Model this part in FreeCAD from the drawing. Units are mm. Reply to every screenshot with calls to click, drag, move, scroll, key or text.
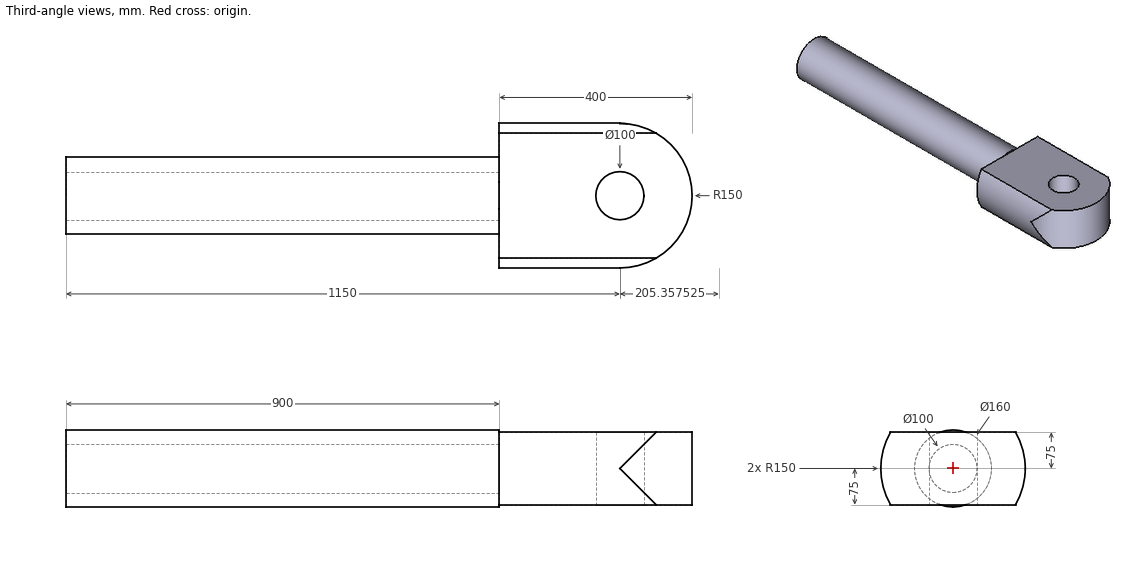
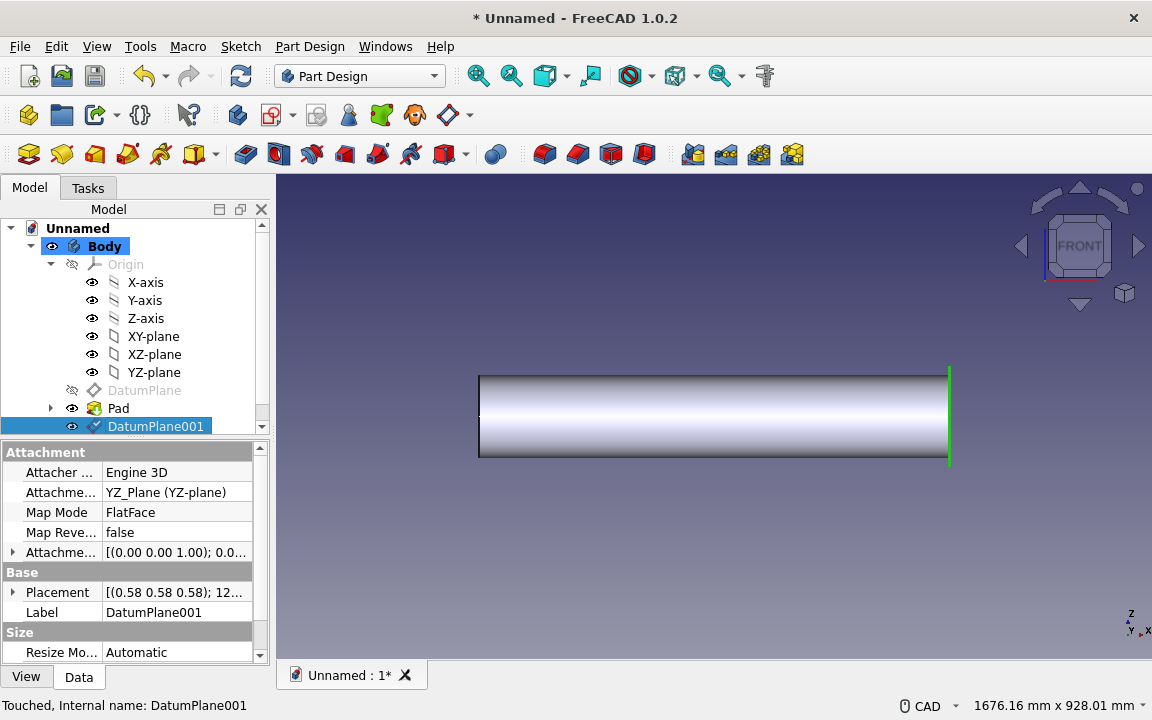
click(270, 116)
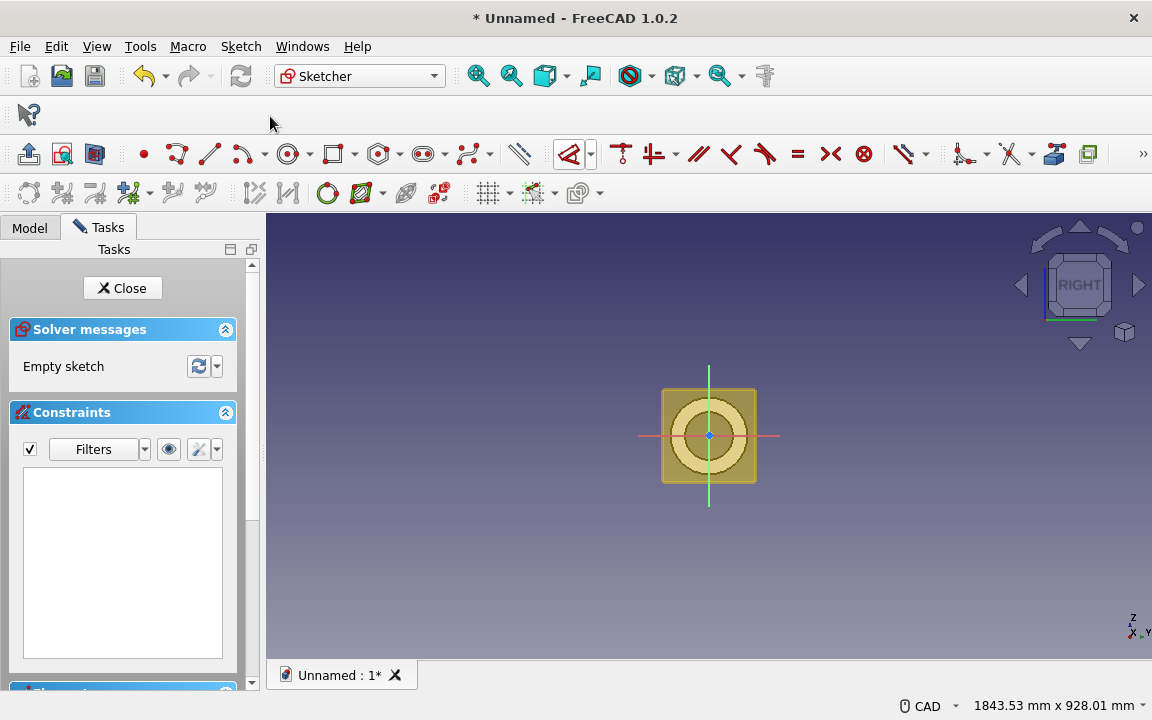
scroll(739, 436, up, 6)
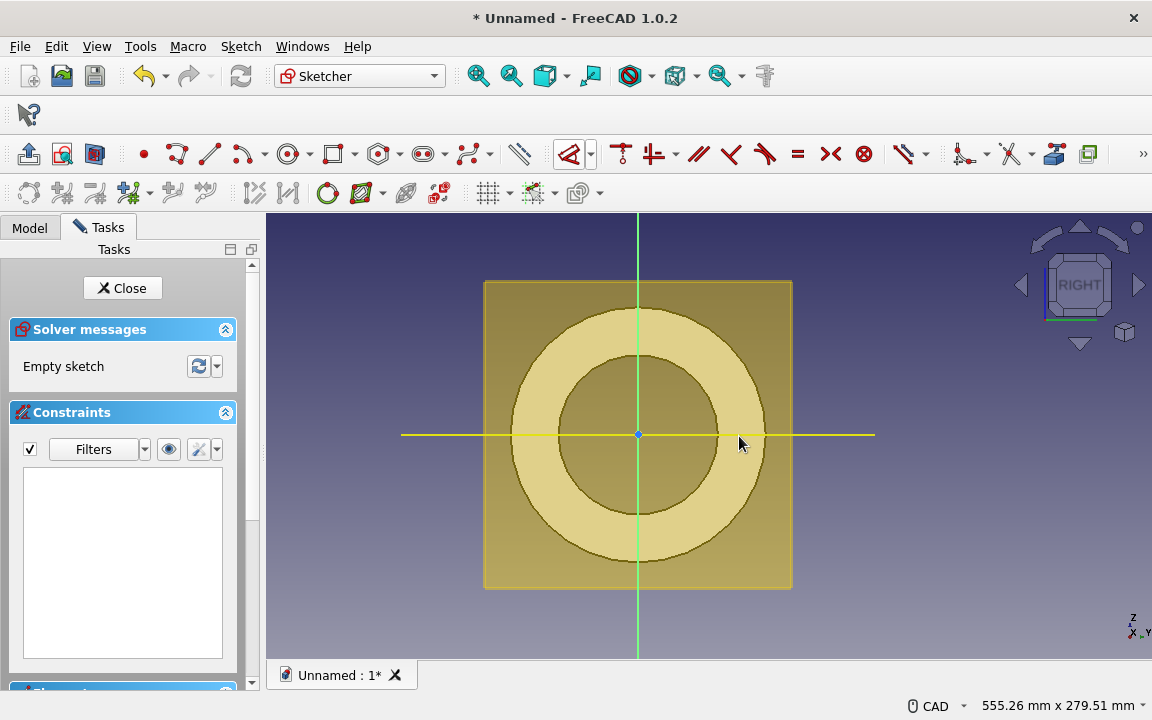
click(210, 154)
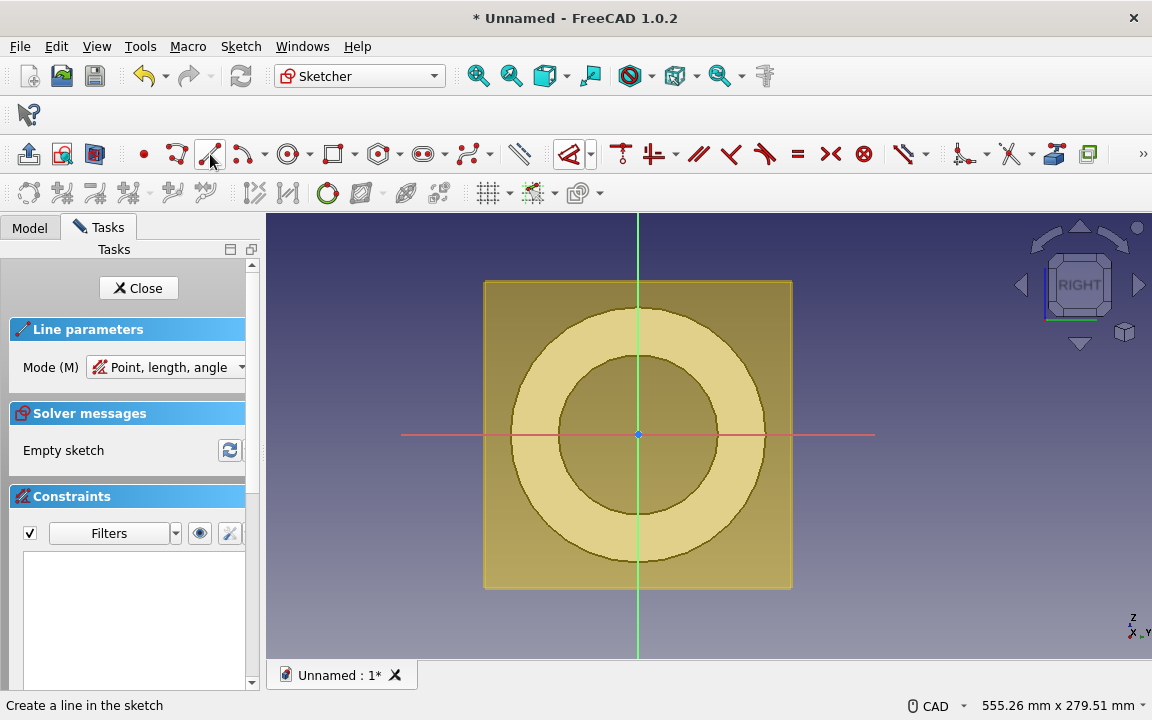
click(845, 315)
click(431, 315)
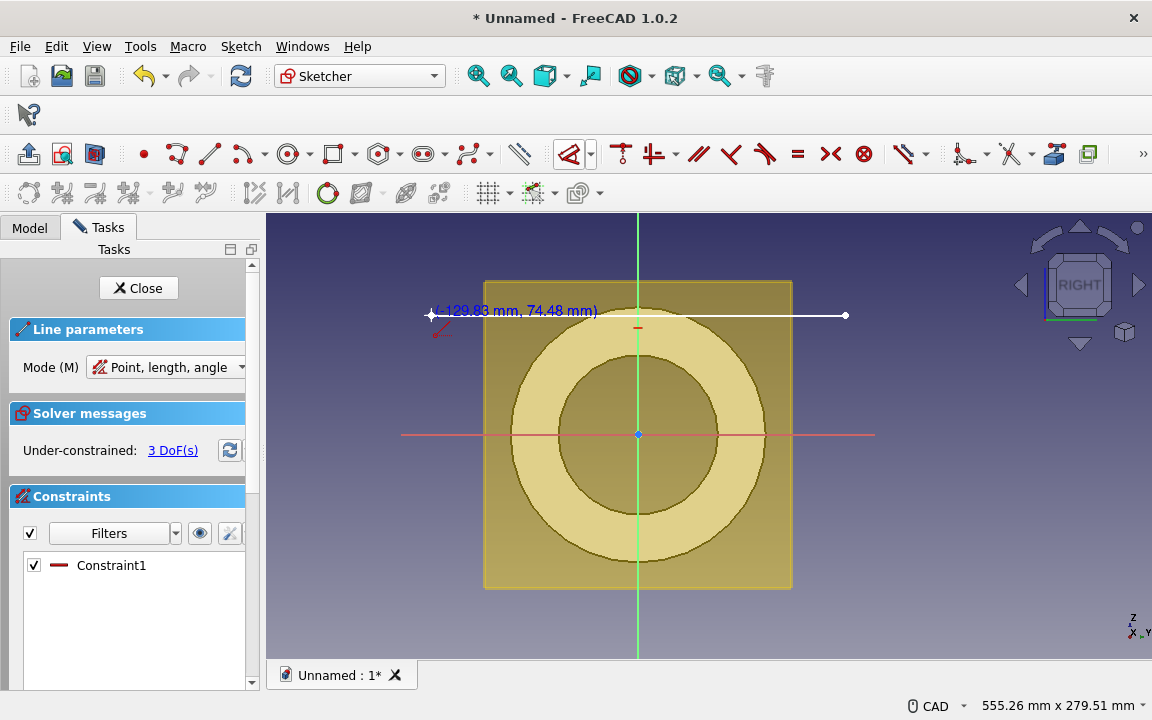
click(431, 555)
click(845, 555)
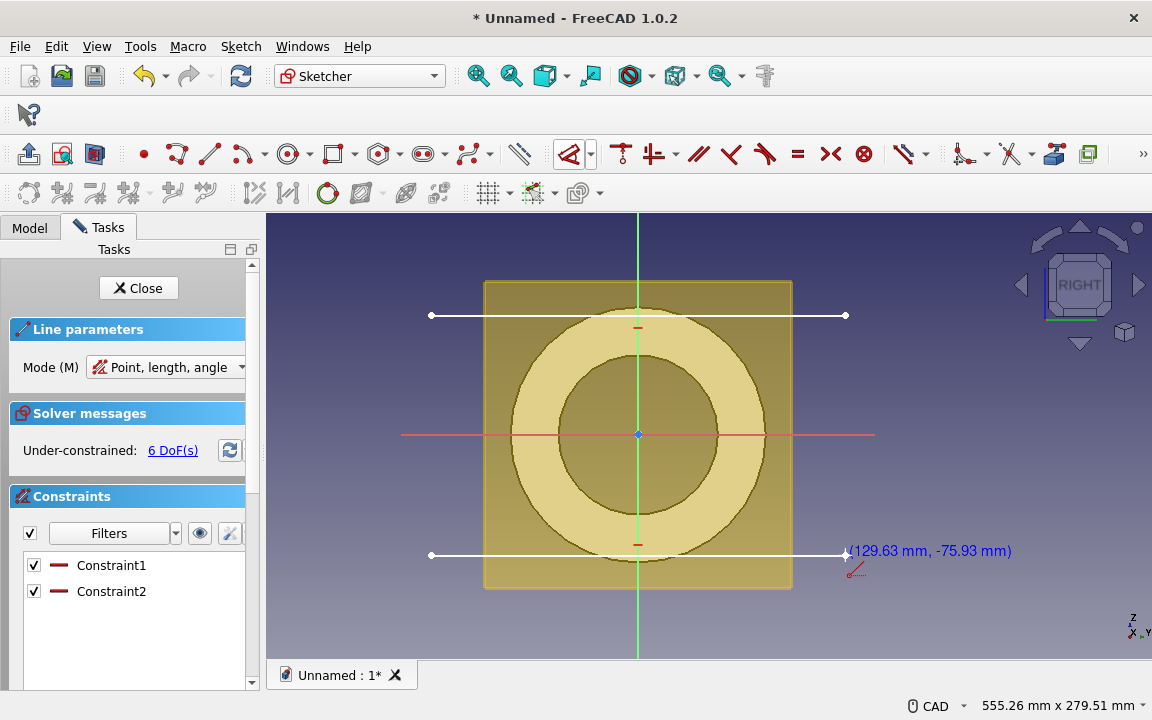
key(g)
key(3)
key(a)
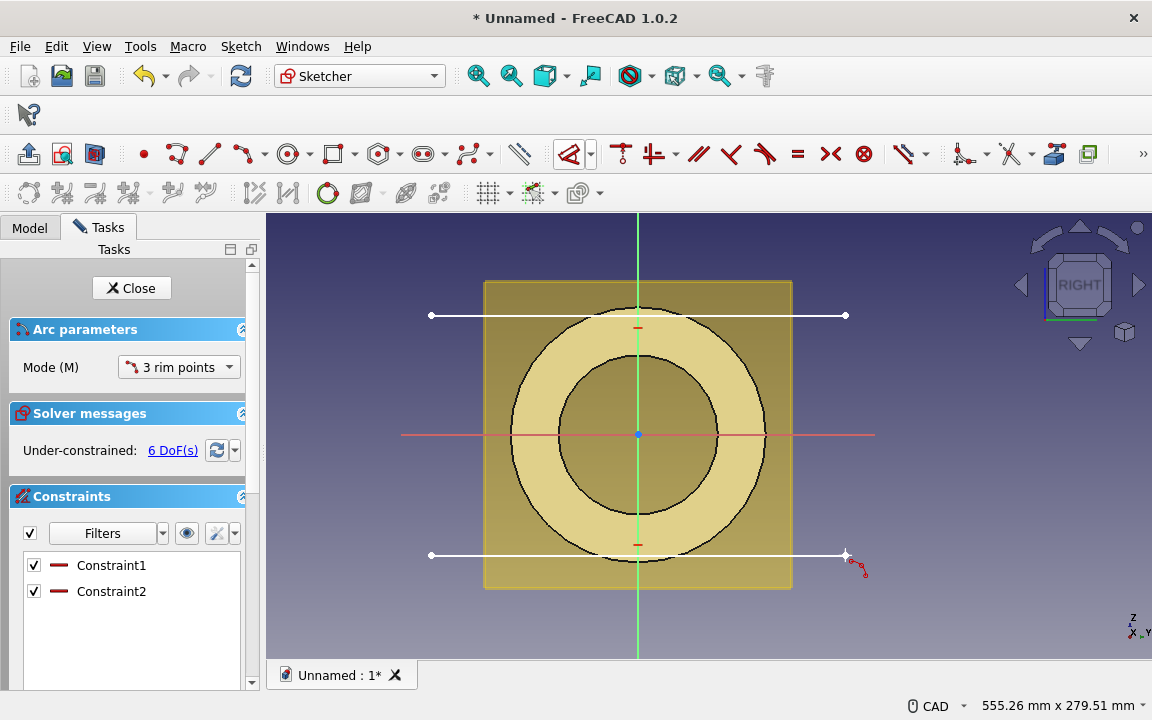
click(431, 316)
click(431, 556)
click(400, 410)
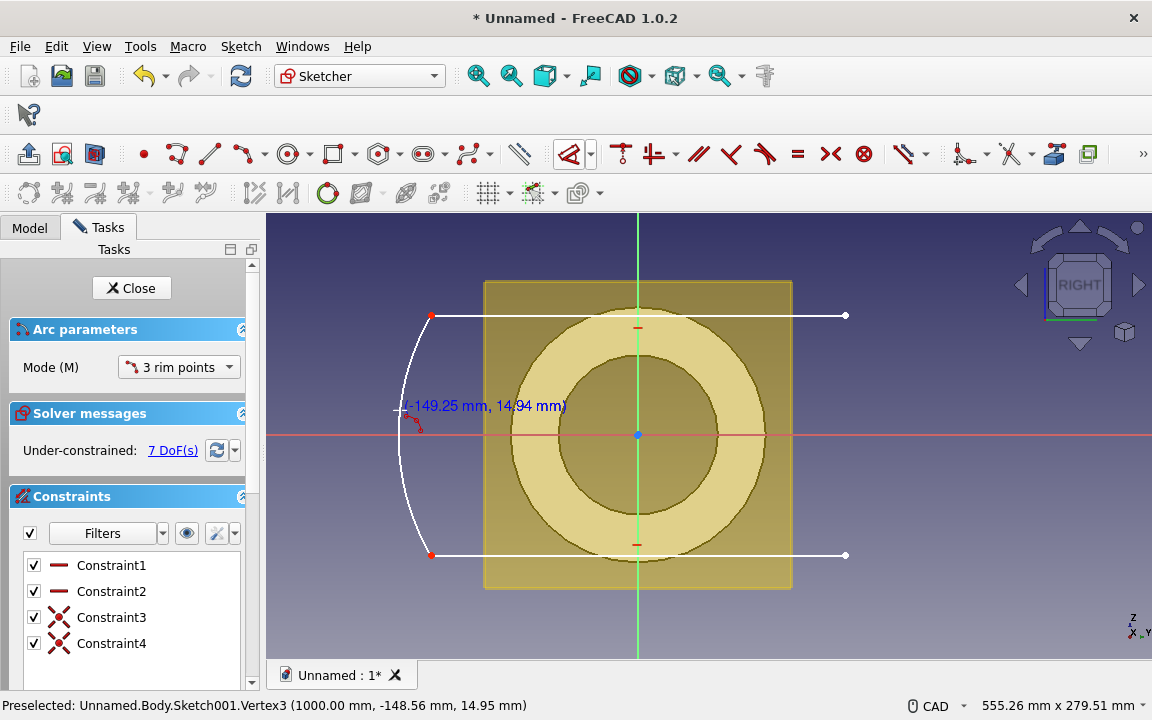
click(845, 556)
click(845, 316)
click(876, 460)
key(Escape)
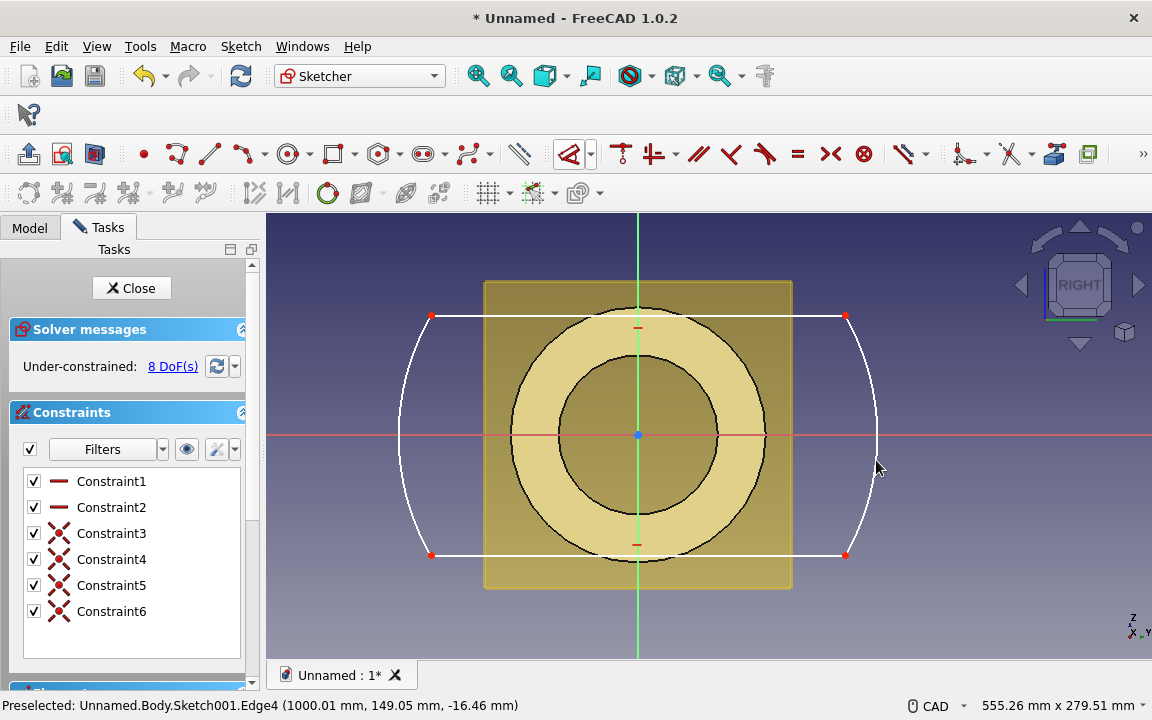
click(404, 386)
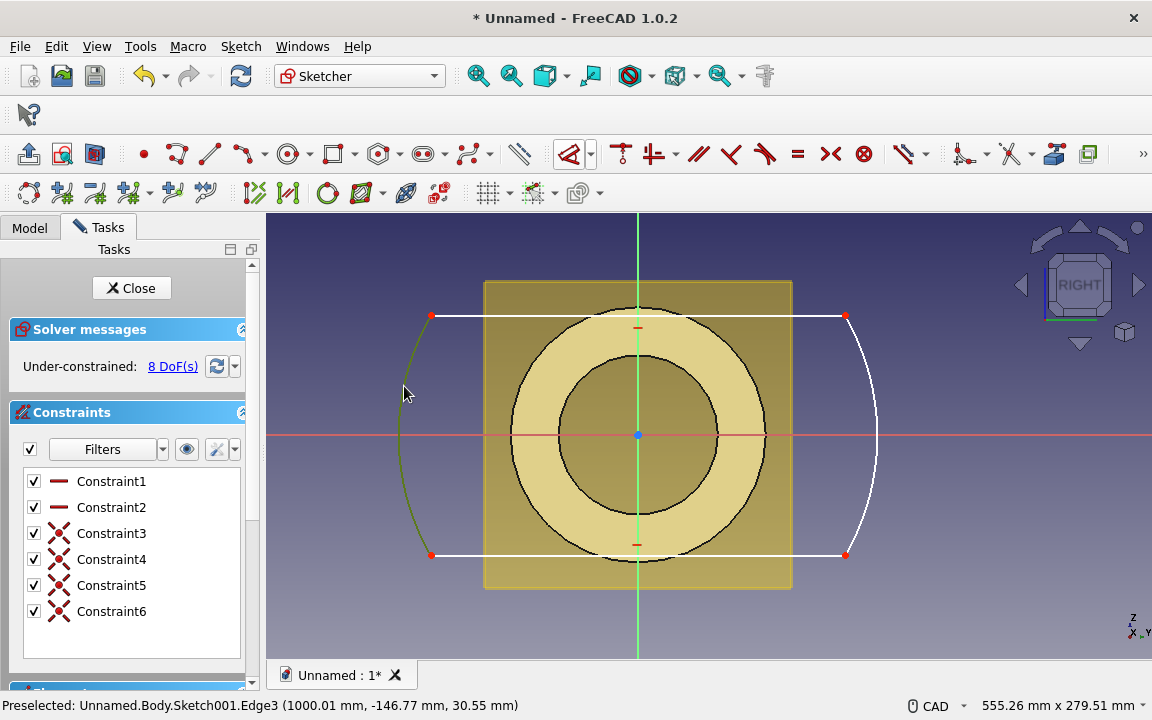
click(872, 486)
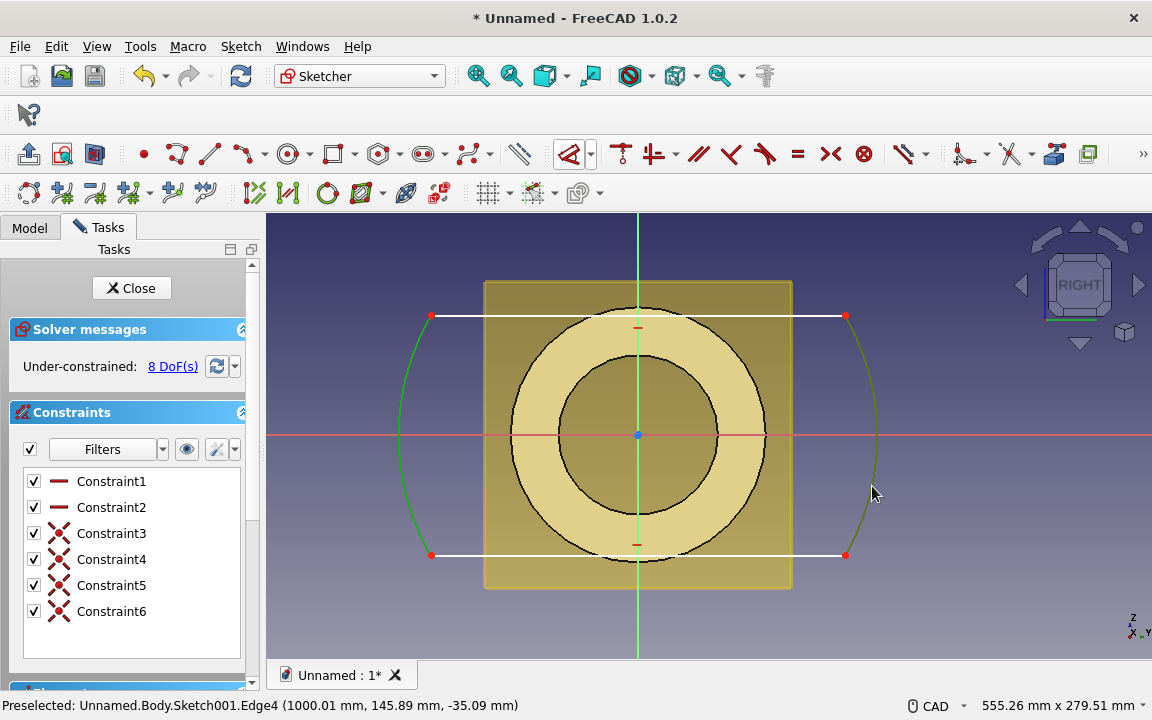
click(621, 154)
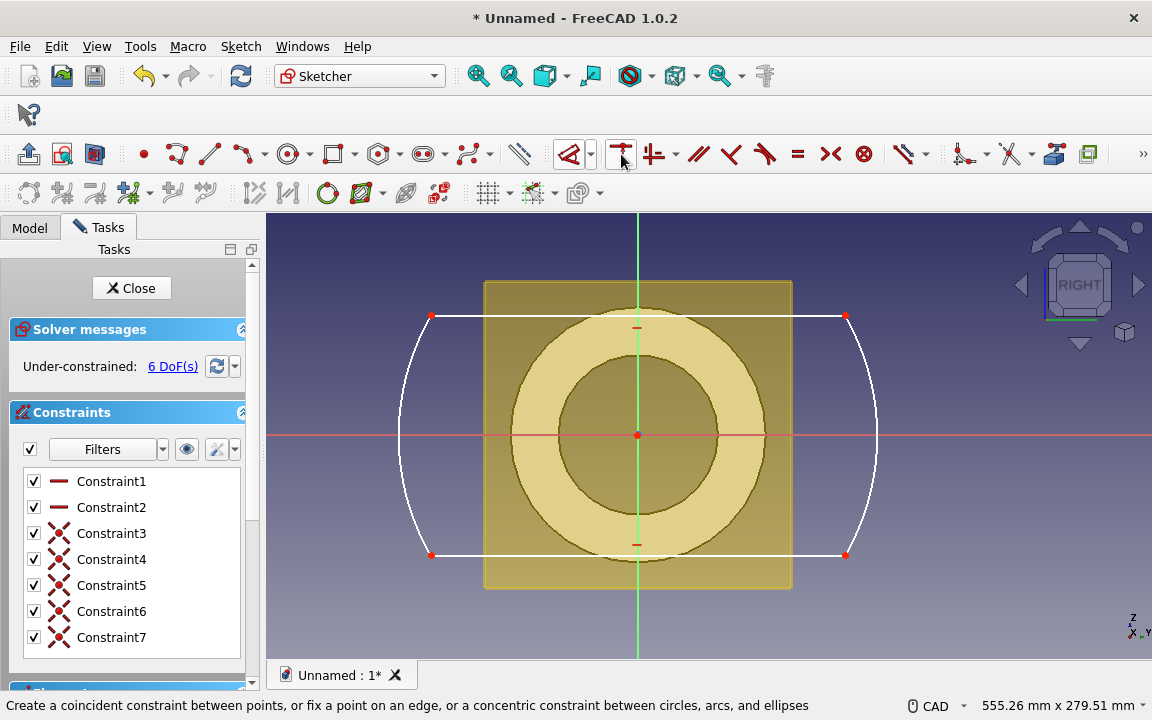
drag(628, 425, 648, 446)